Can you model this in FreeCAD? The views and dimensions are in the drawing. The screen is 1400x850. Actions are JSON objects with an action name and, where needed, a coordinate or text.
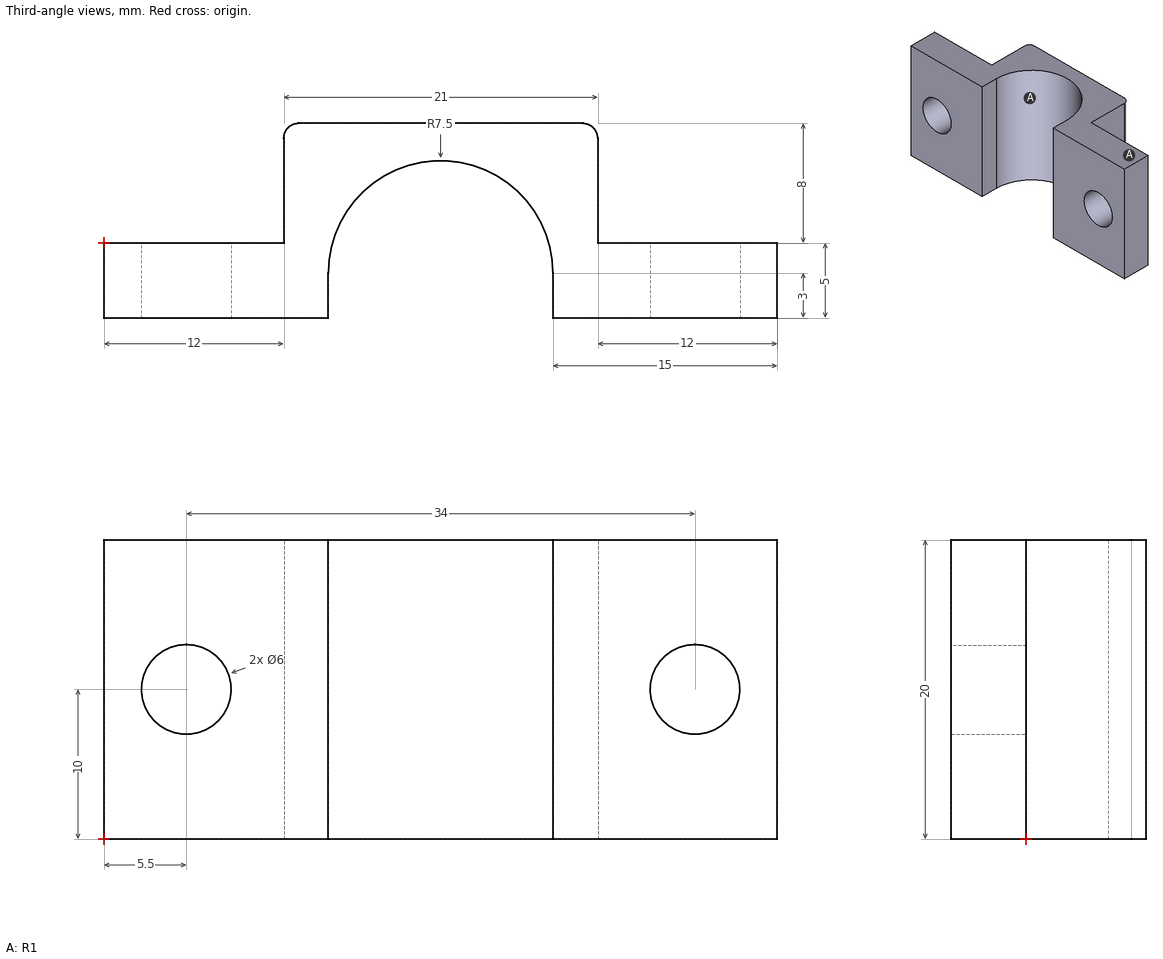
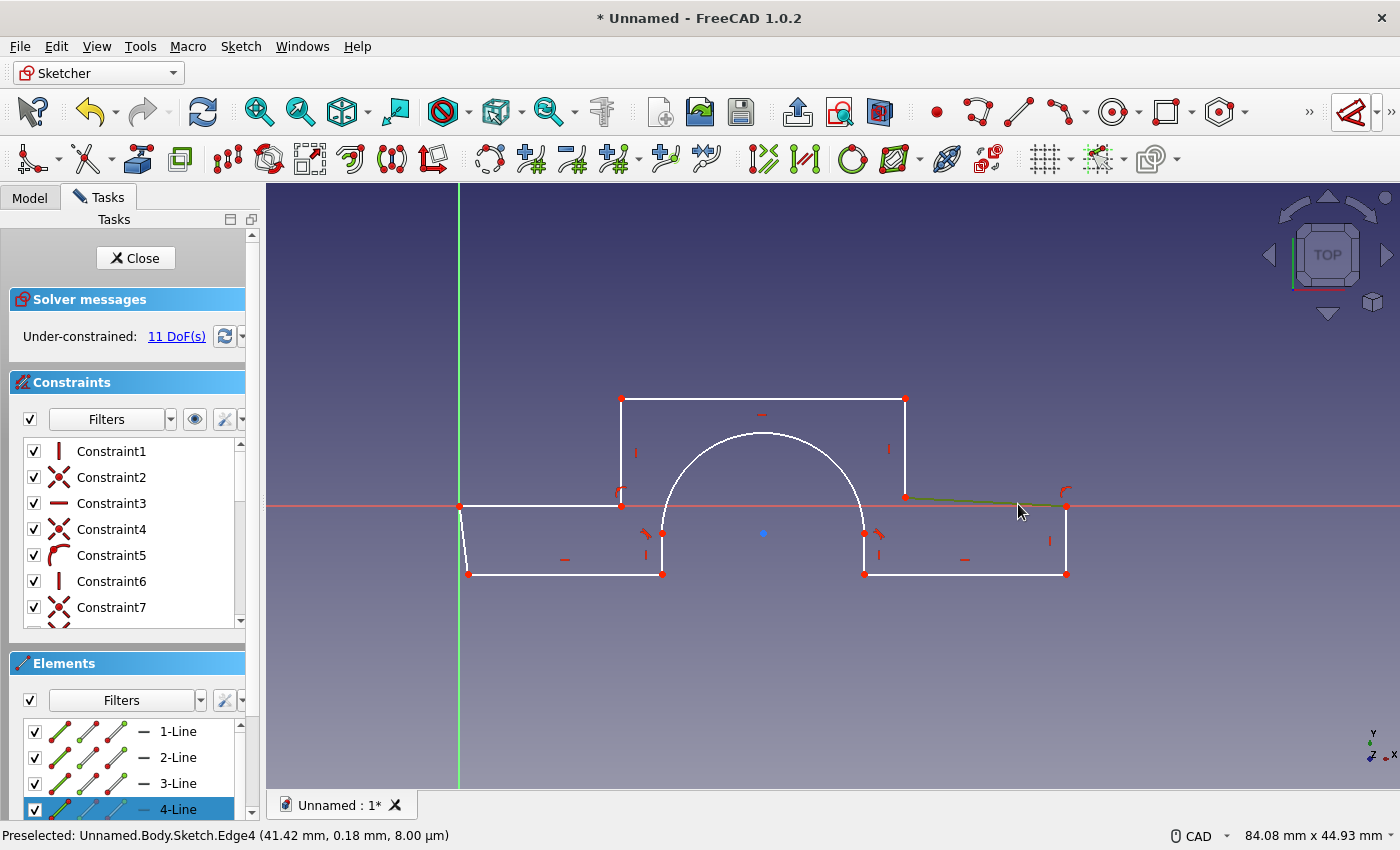
{"action": "key", "text": "h"}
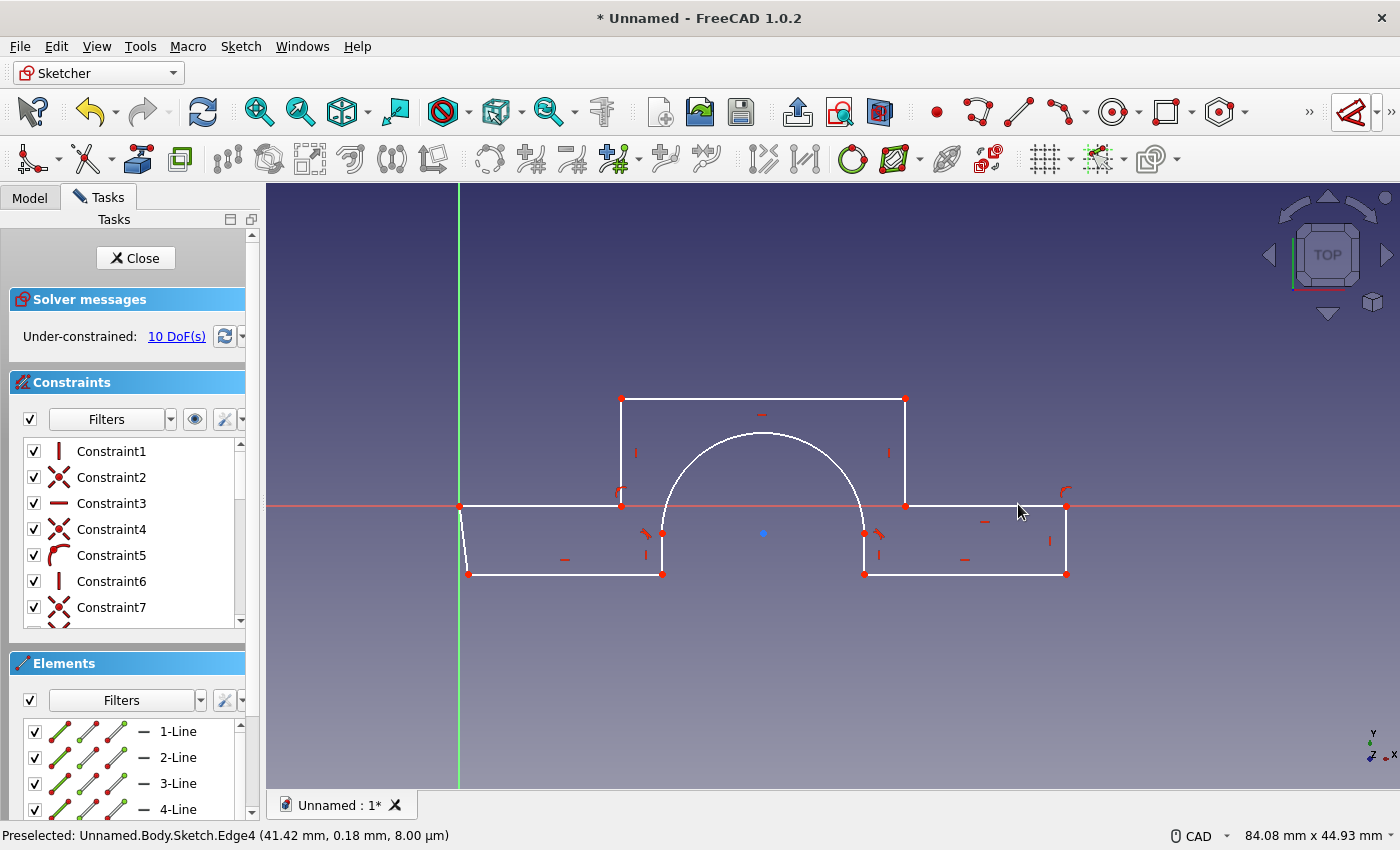
{"action": "left_click", "coordinate": [462, 527]}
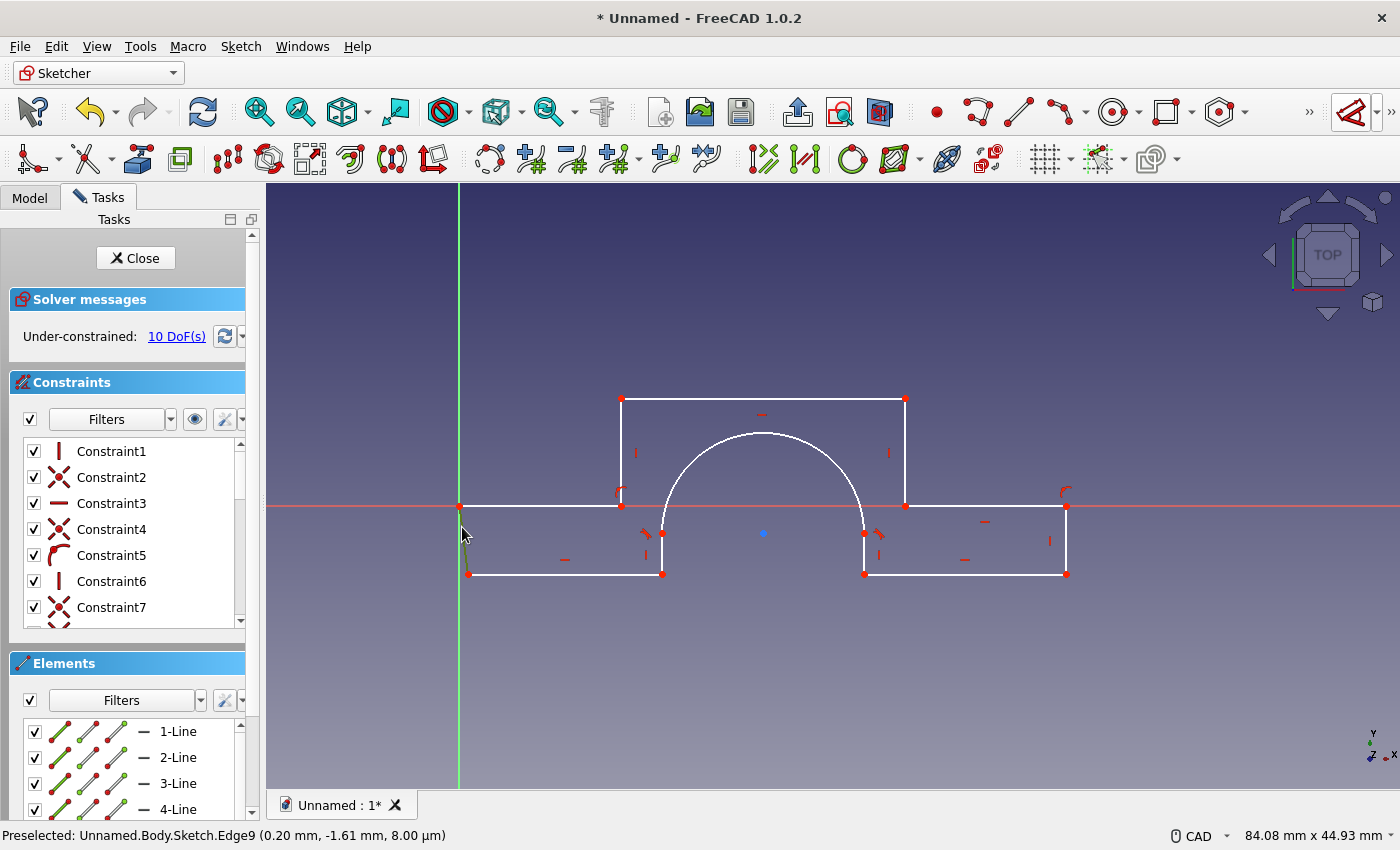
{"action": "key", "text": "v"}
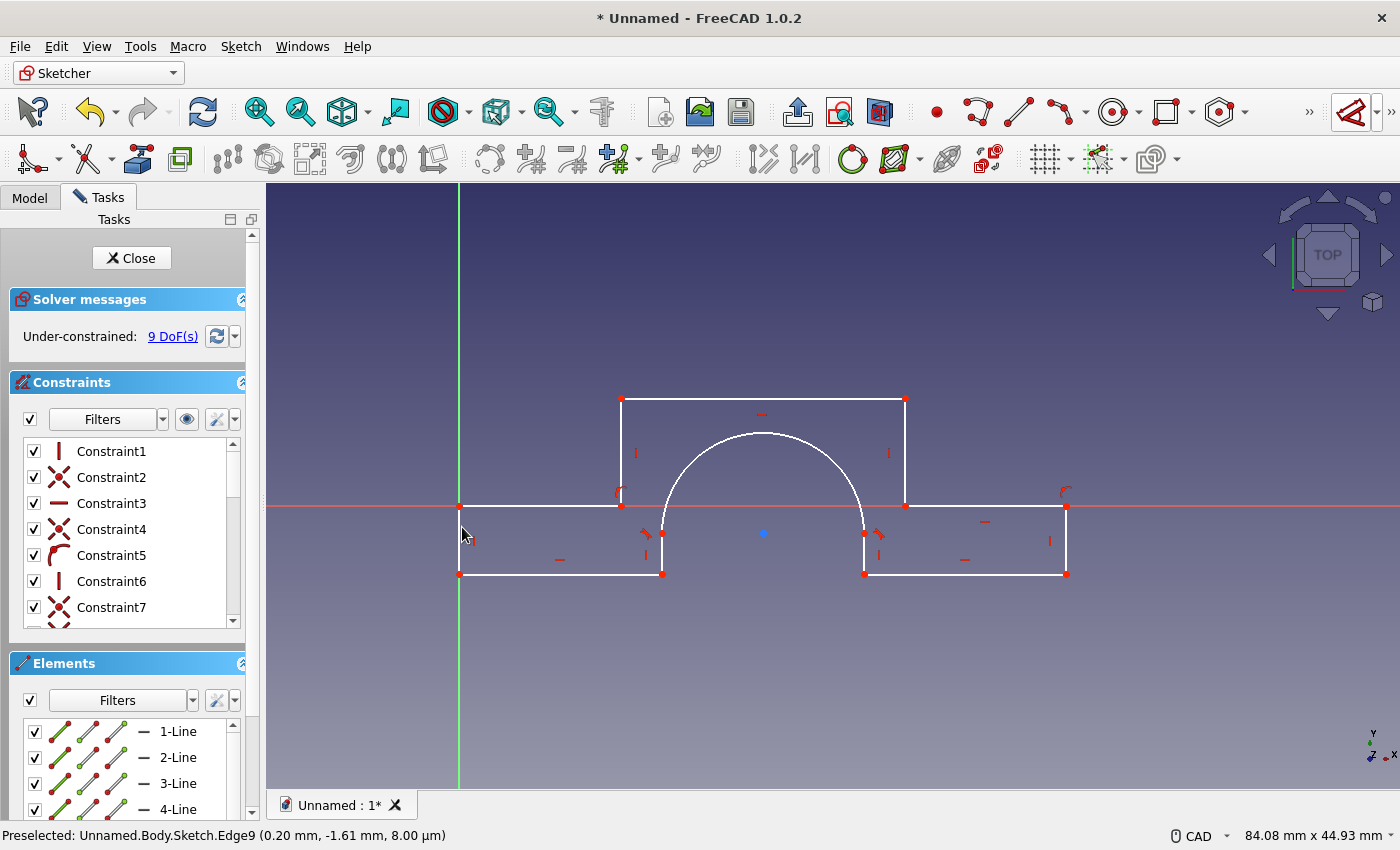
{"action": "left_click", "coordinate": [822, 452]}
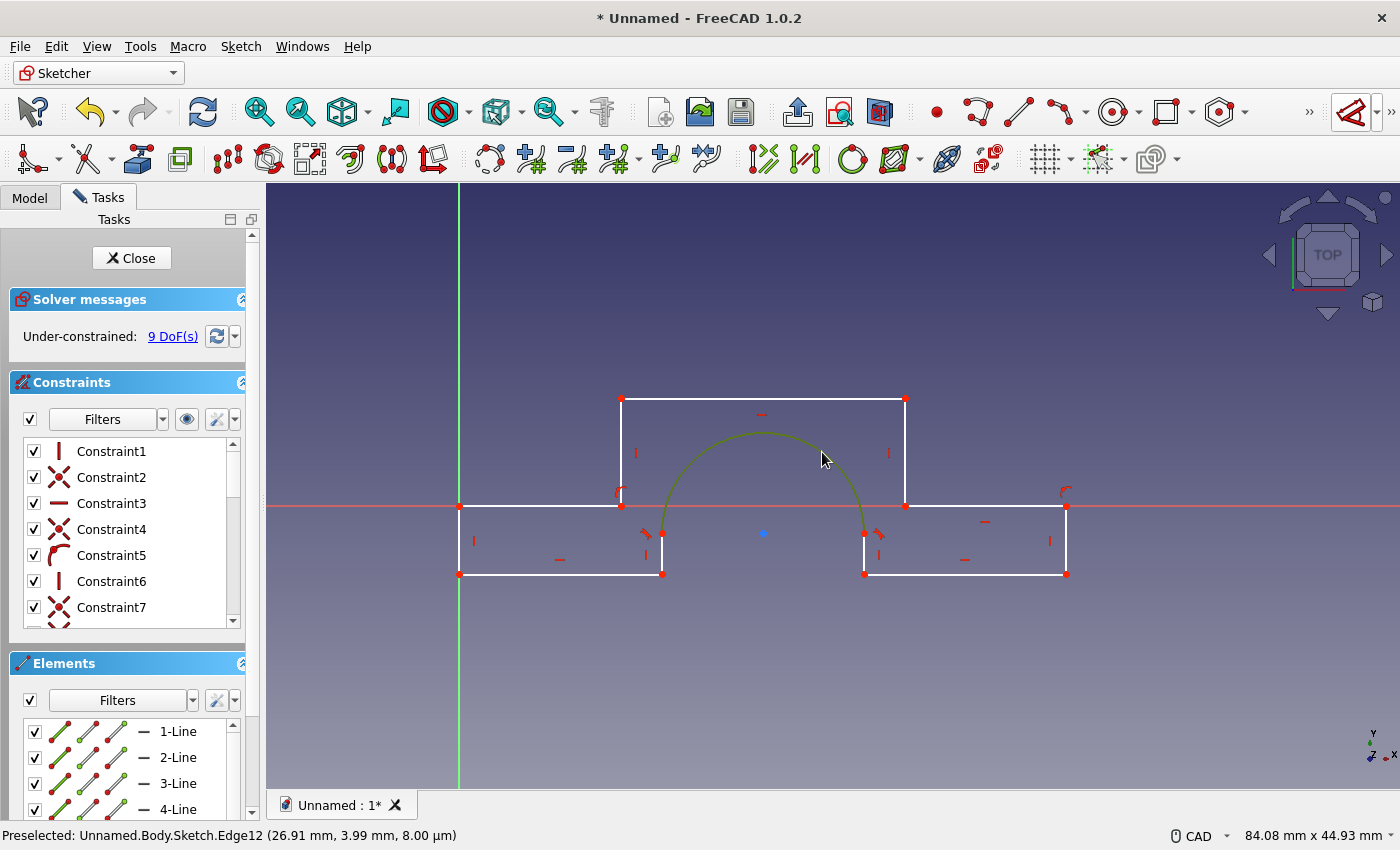
{"action": "key", "text": "k r"}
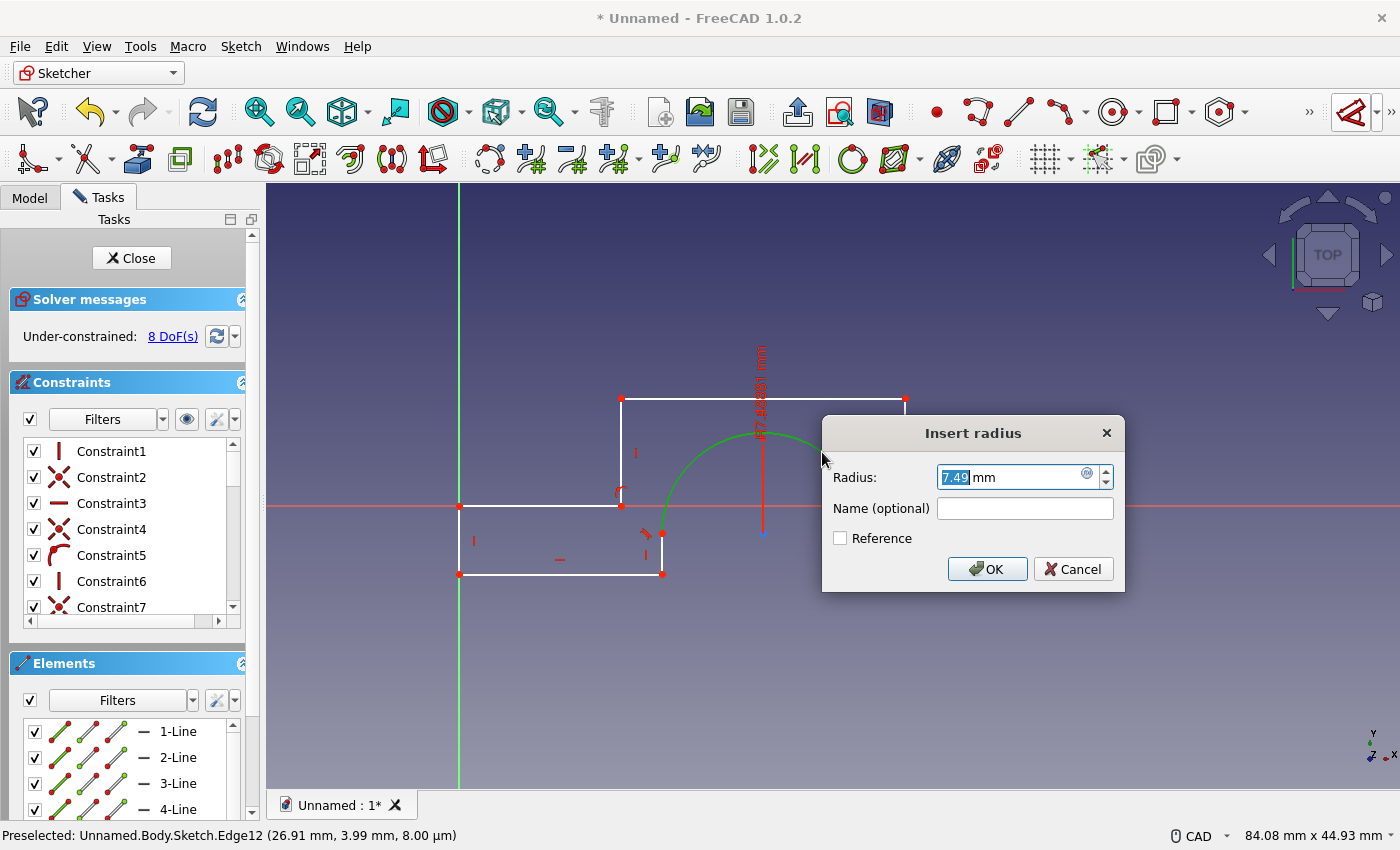
{"action": "type", "text": "7.5"}
{"action": "key", "text": "Return"}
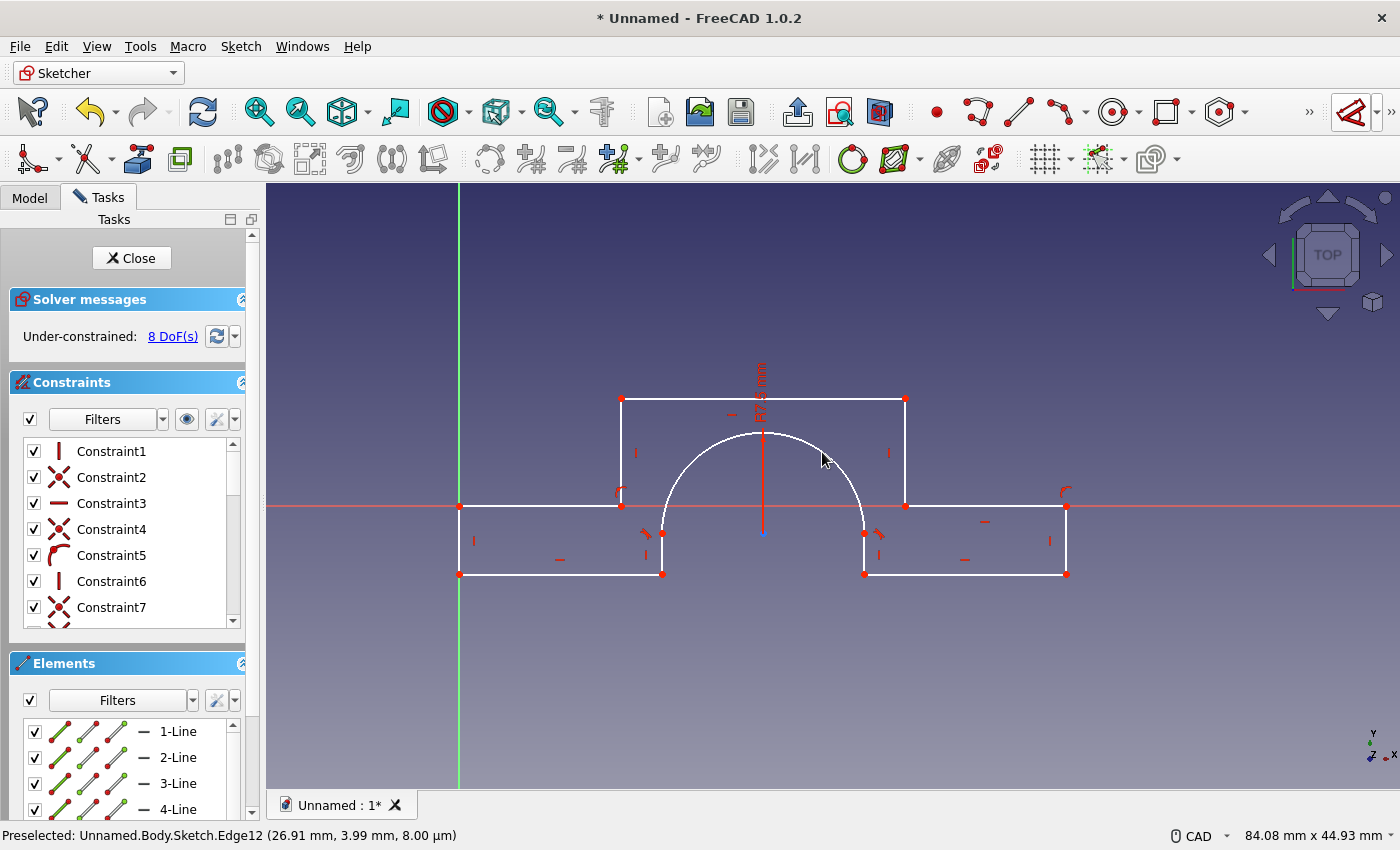
{"action": "left_click", "coordinate": [864, 546]}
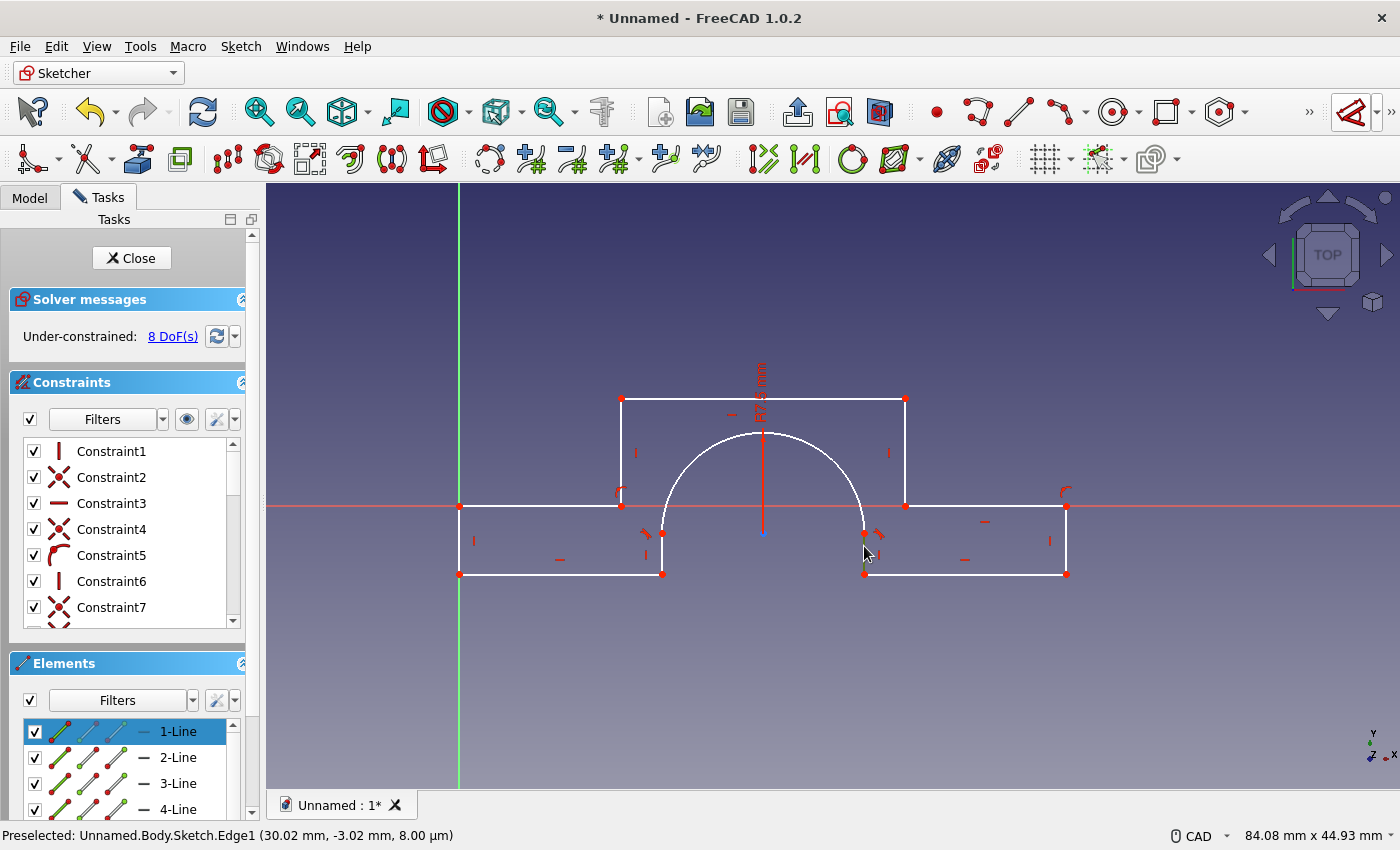
{"action": "key", "text": "i"}